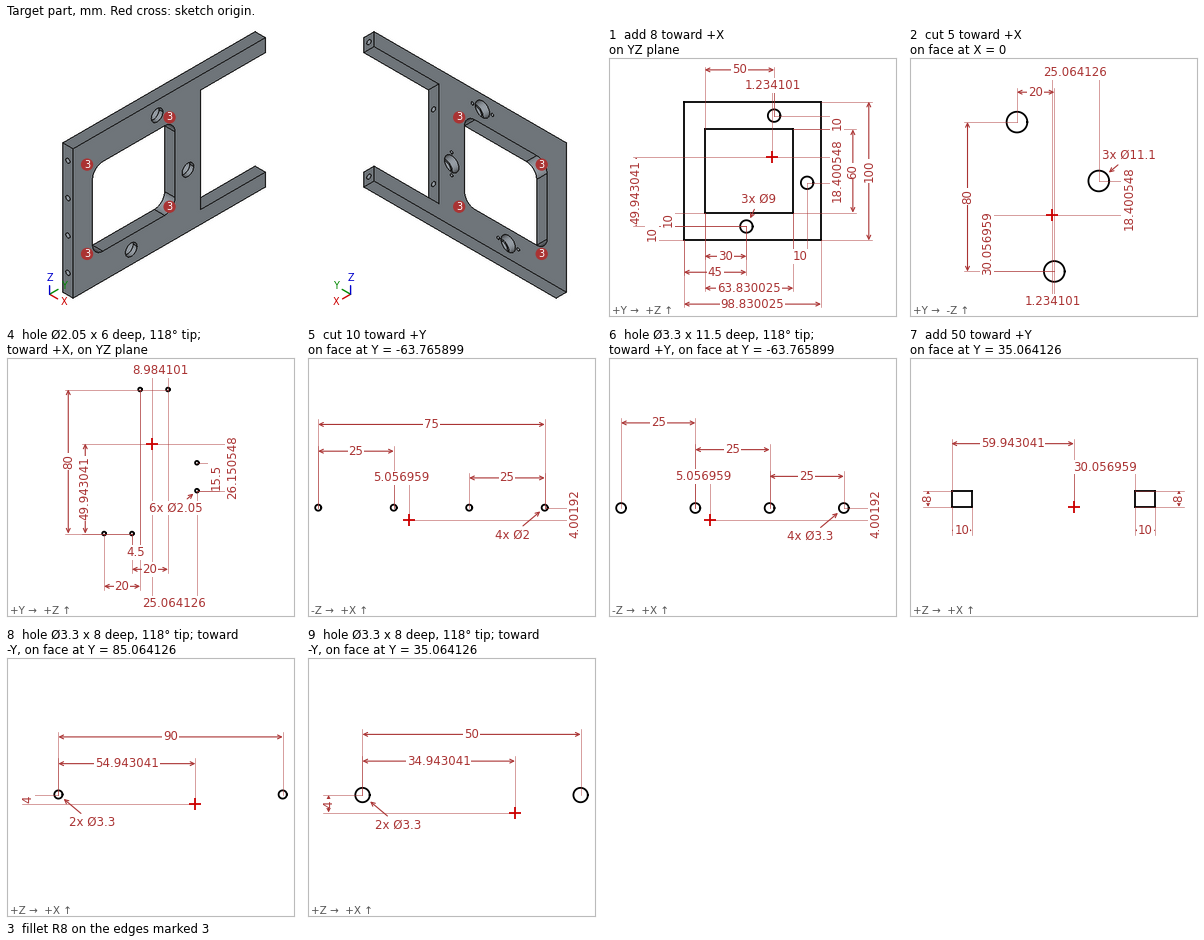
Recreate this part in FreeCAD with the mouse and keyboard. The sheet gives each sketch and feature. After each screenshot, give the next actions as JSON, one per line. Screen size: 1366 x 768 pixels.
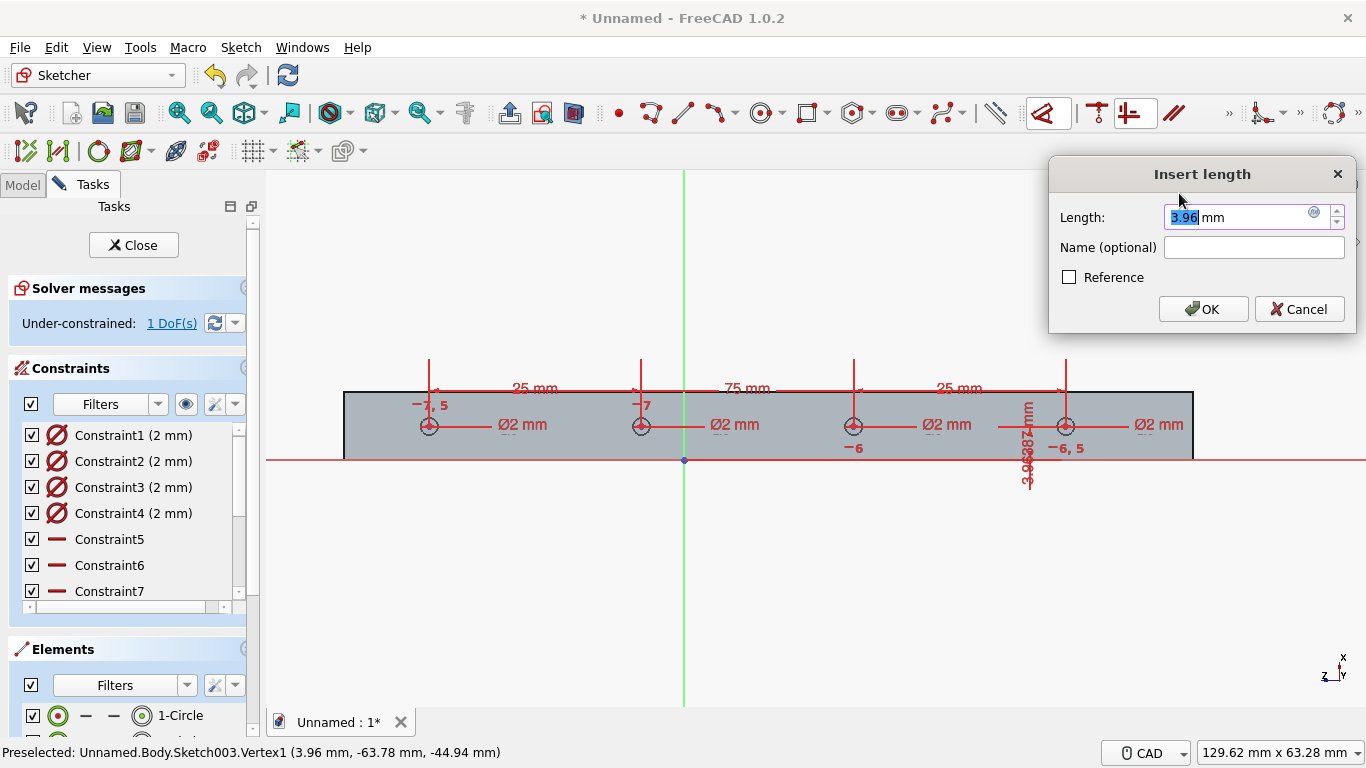
{"action": "type", "text": "4.00192"}
{"action": "key", "text": "Return"}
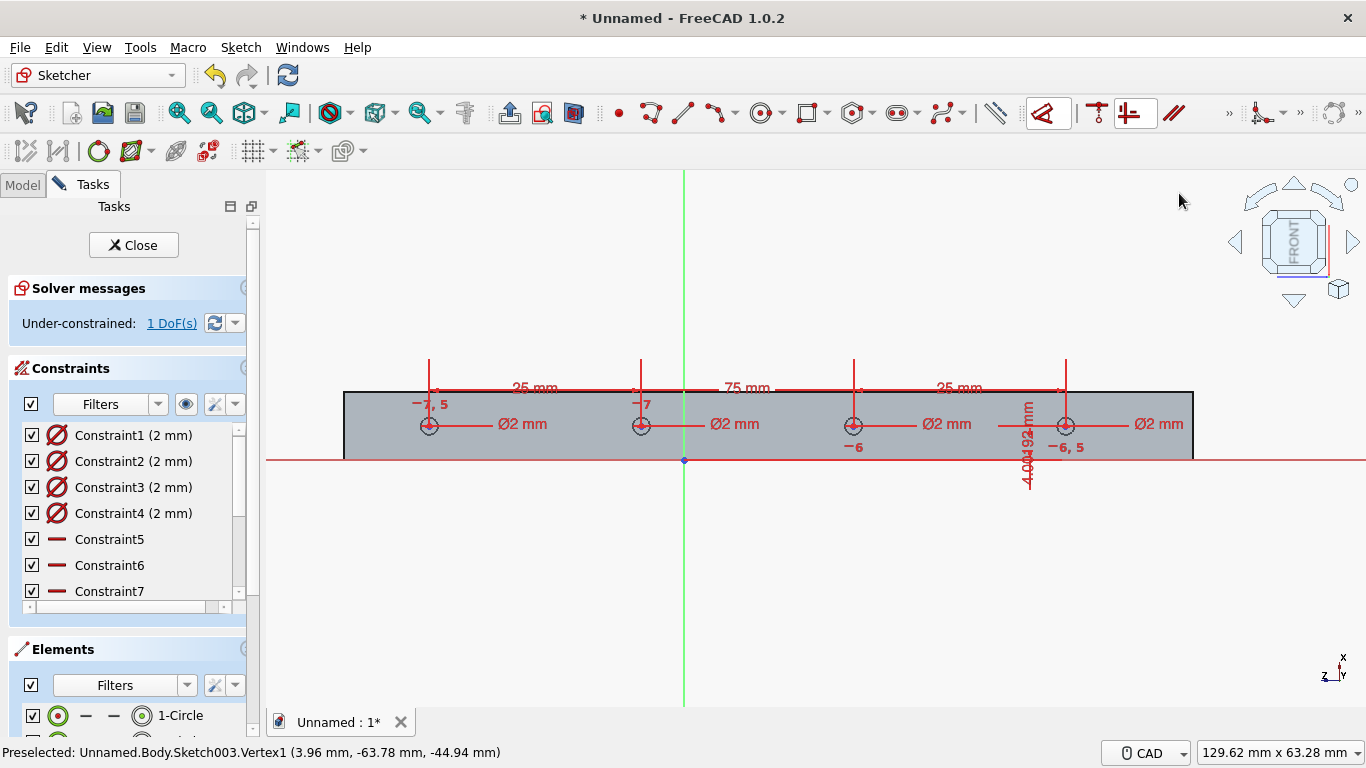
{"action": "left_click", "coordinate": [641, 426]}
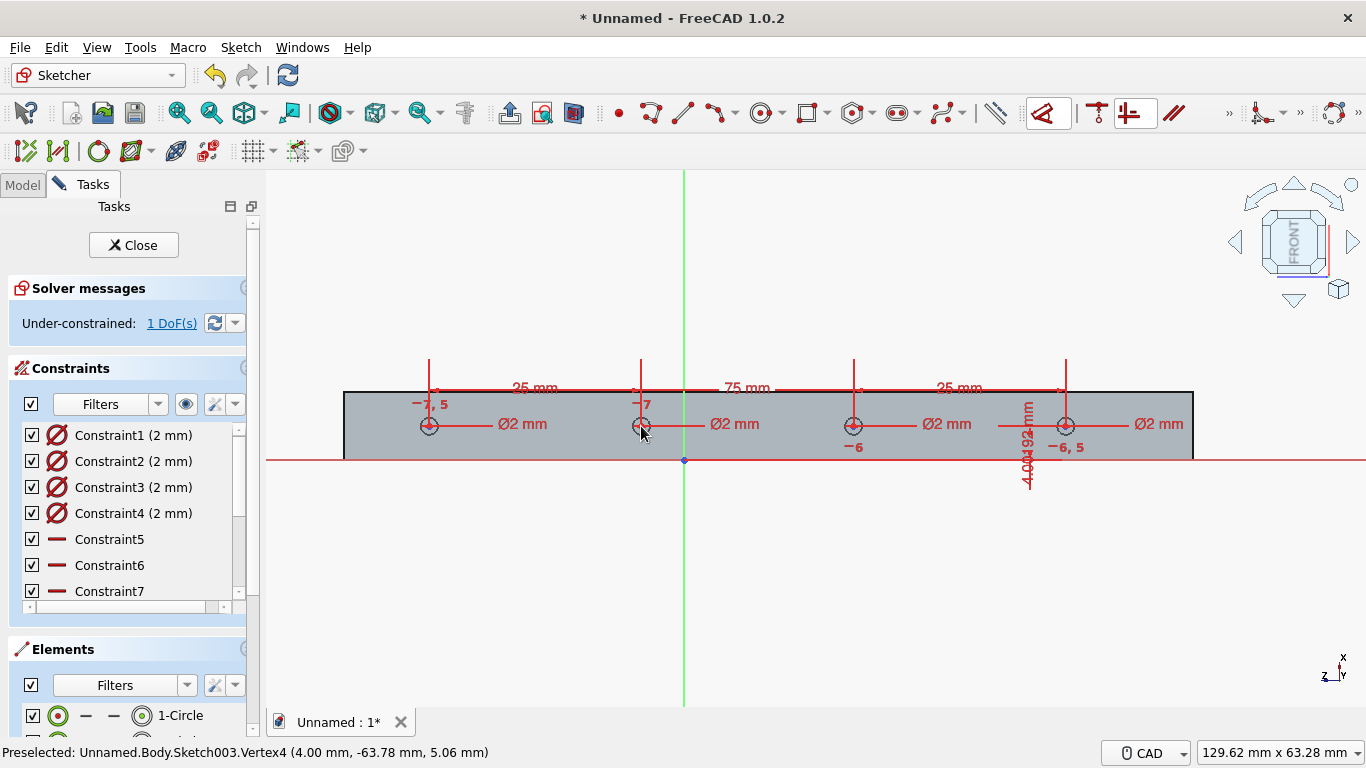
{"action": "key", "text": "l"}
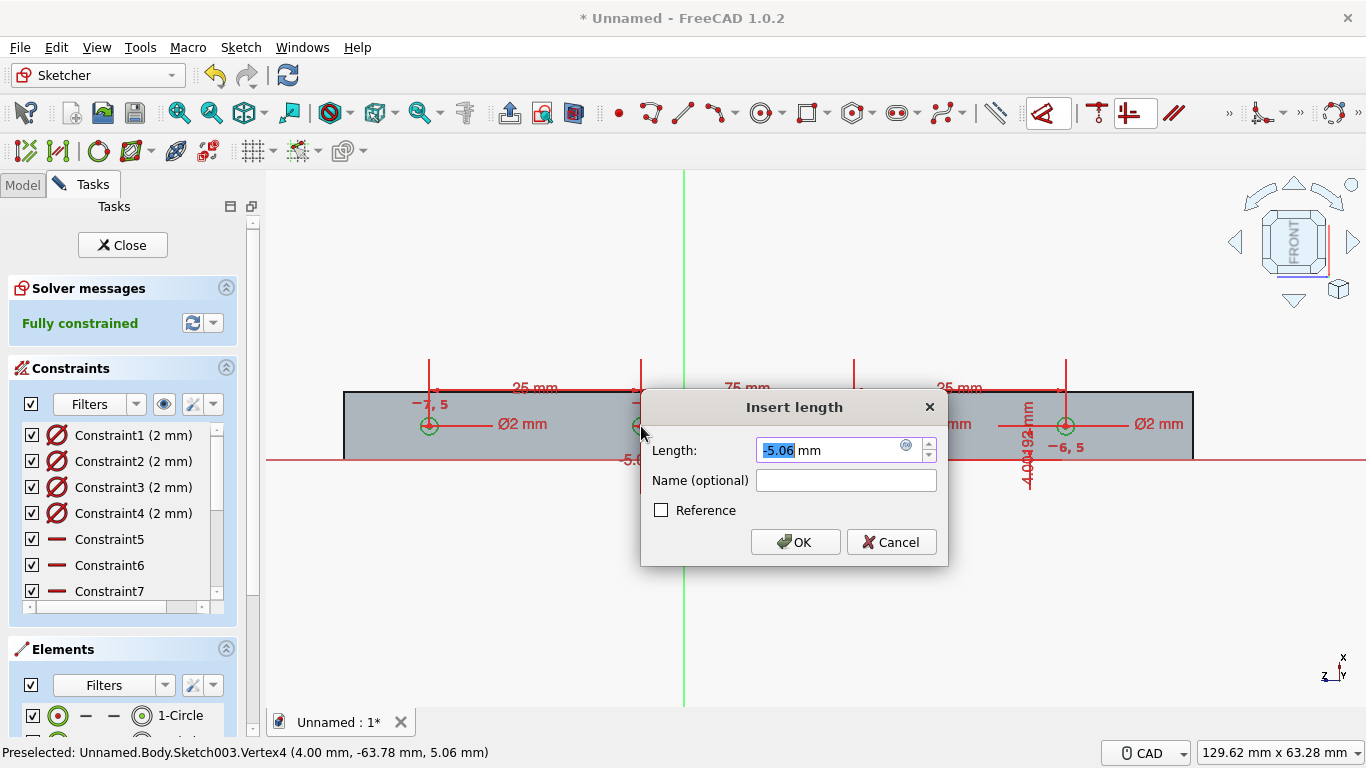
{"action": "type", "text": "-5.056959"}
{"action": "key", "text": "Return"}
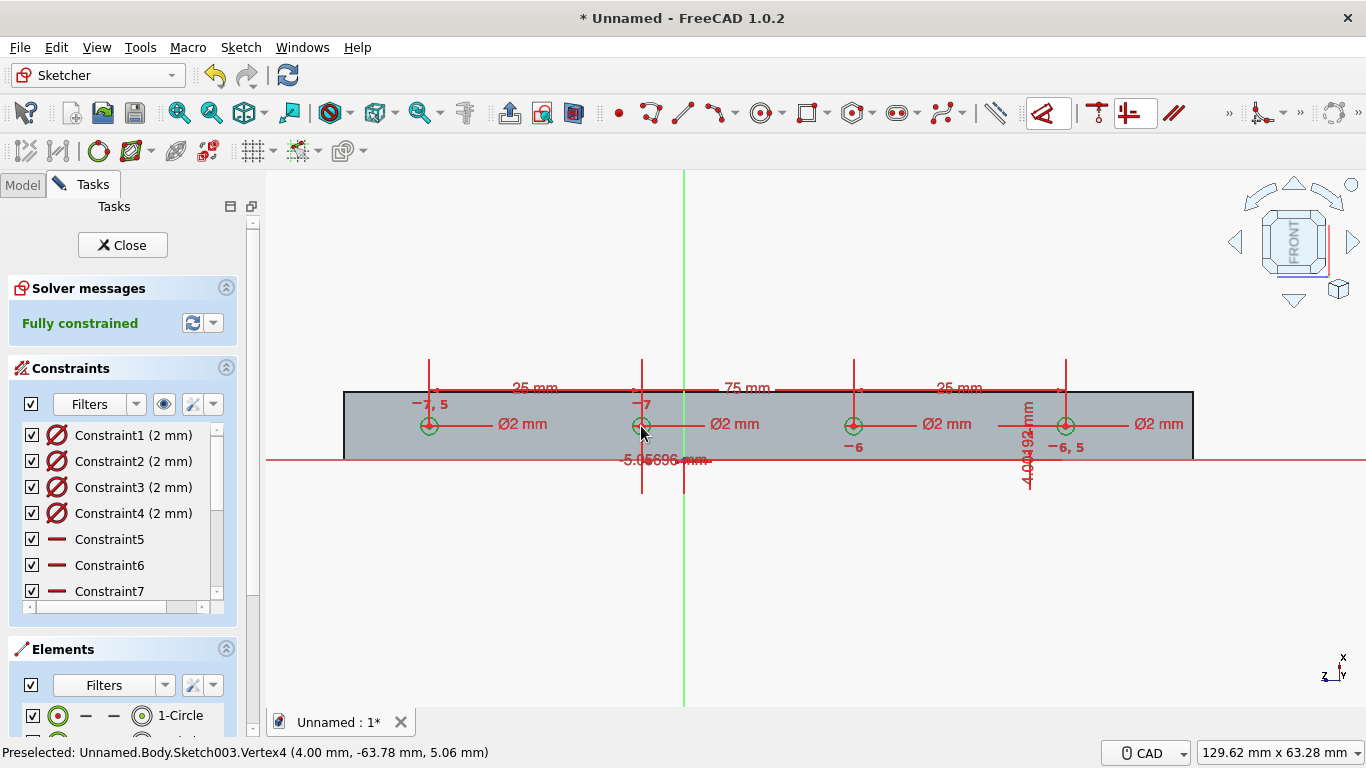
{"action": "left_click", "coordinate": [123, 245]}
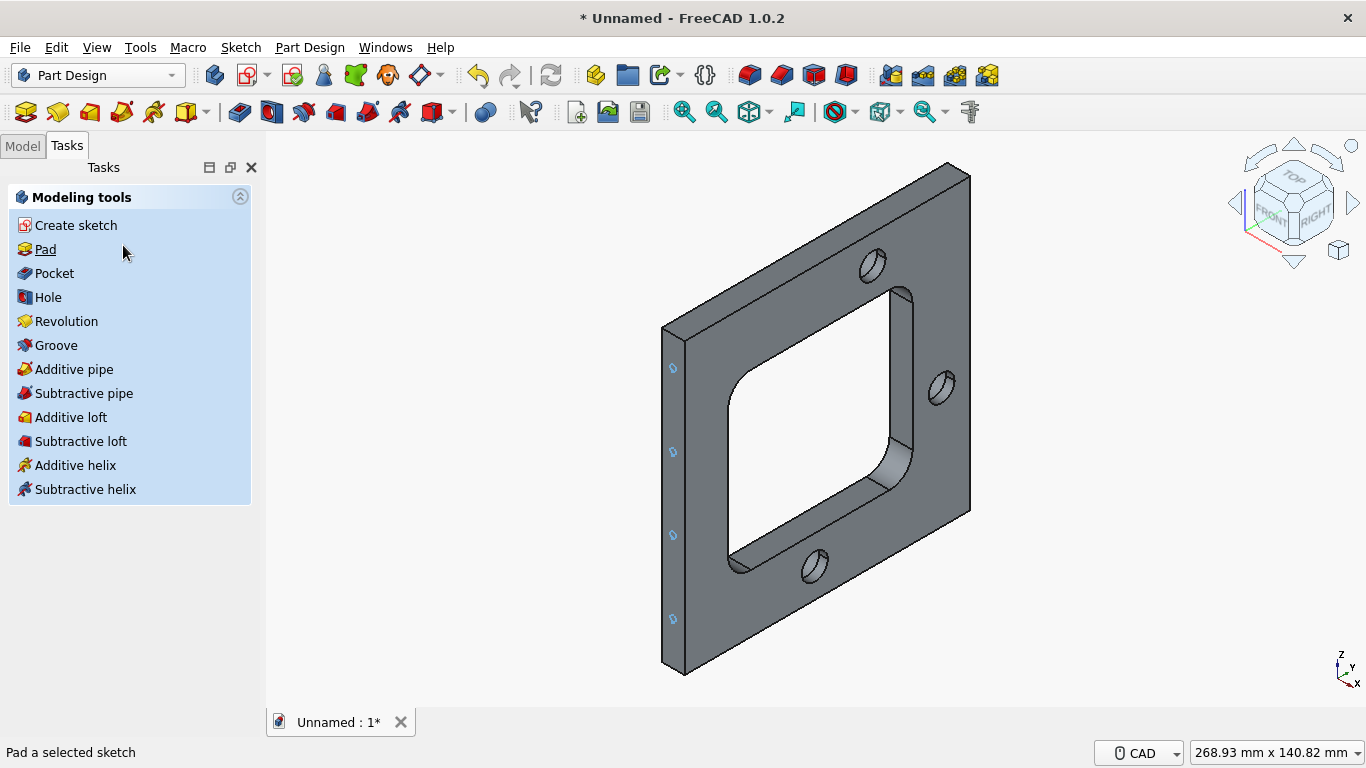
{"action": "left_click", "coordinate": [240, 112]}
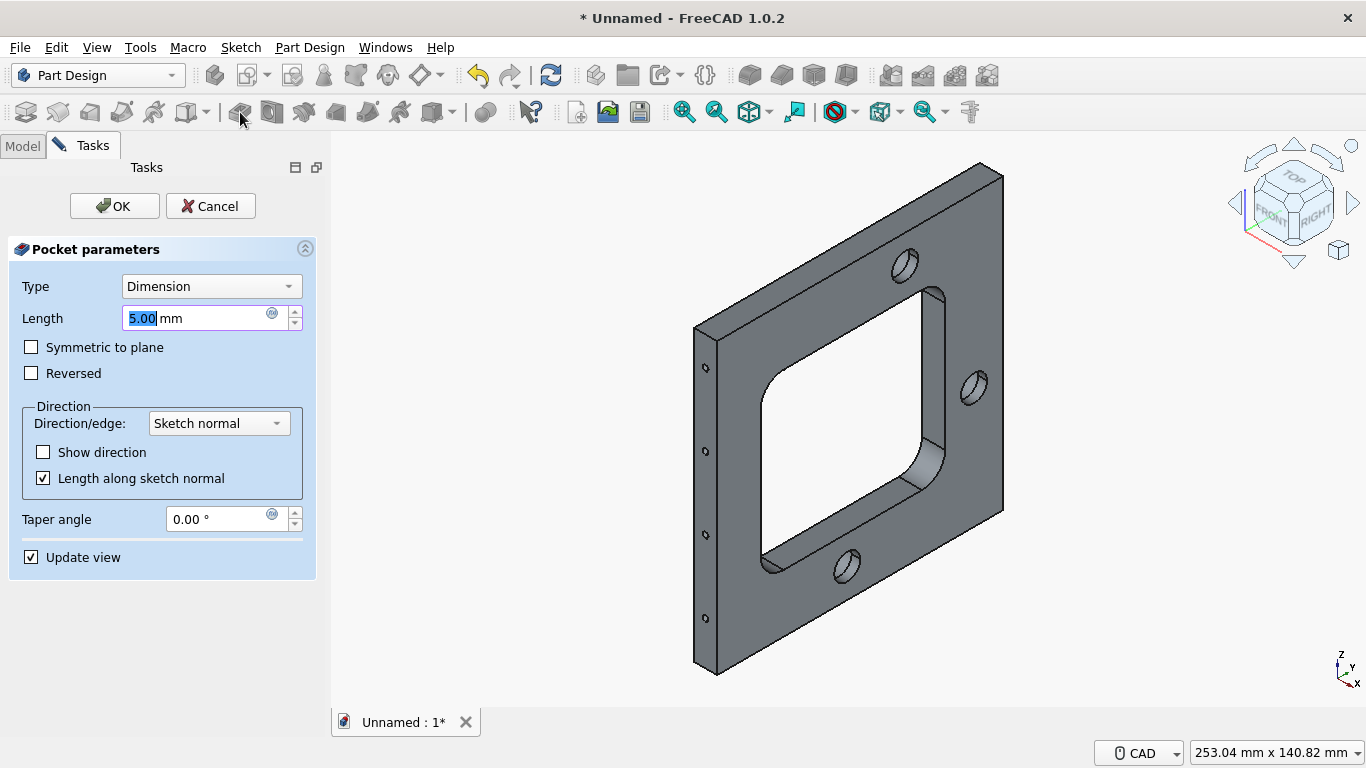
{"action": "type", "text": "10"}
{"action": "key", "text": "Tab"}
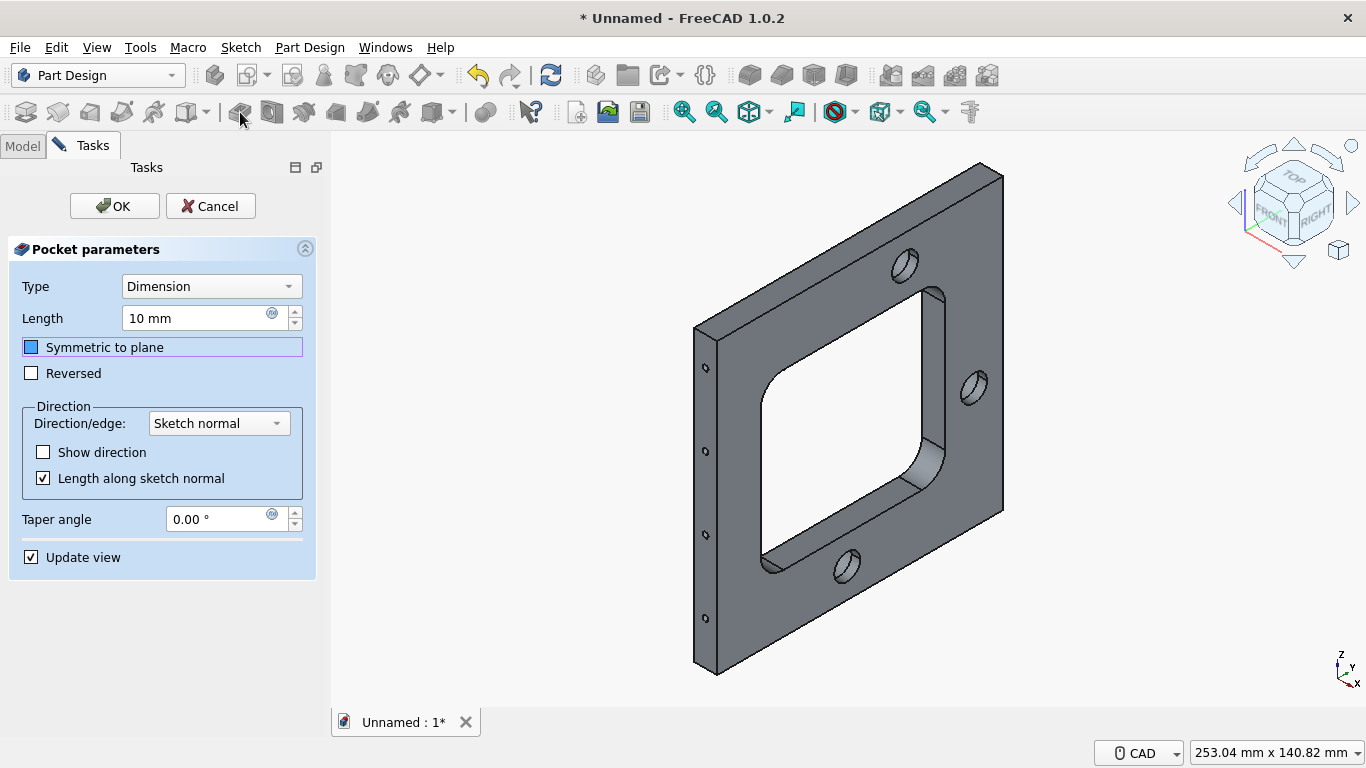
{"action": "left_click", "coordinate": [115, 206]}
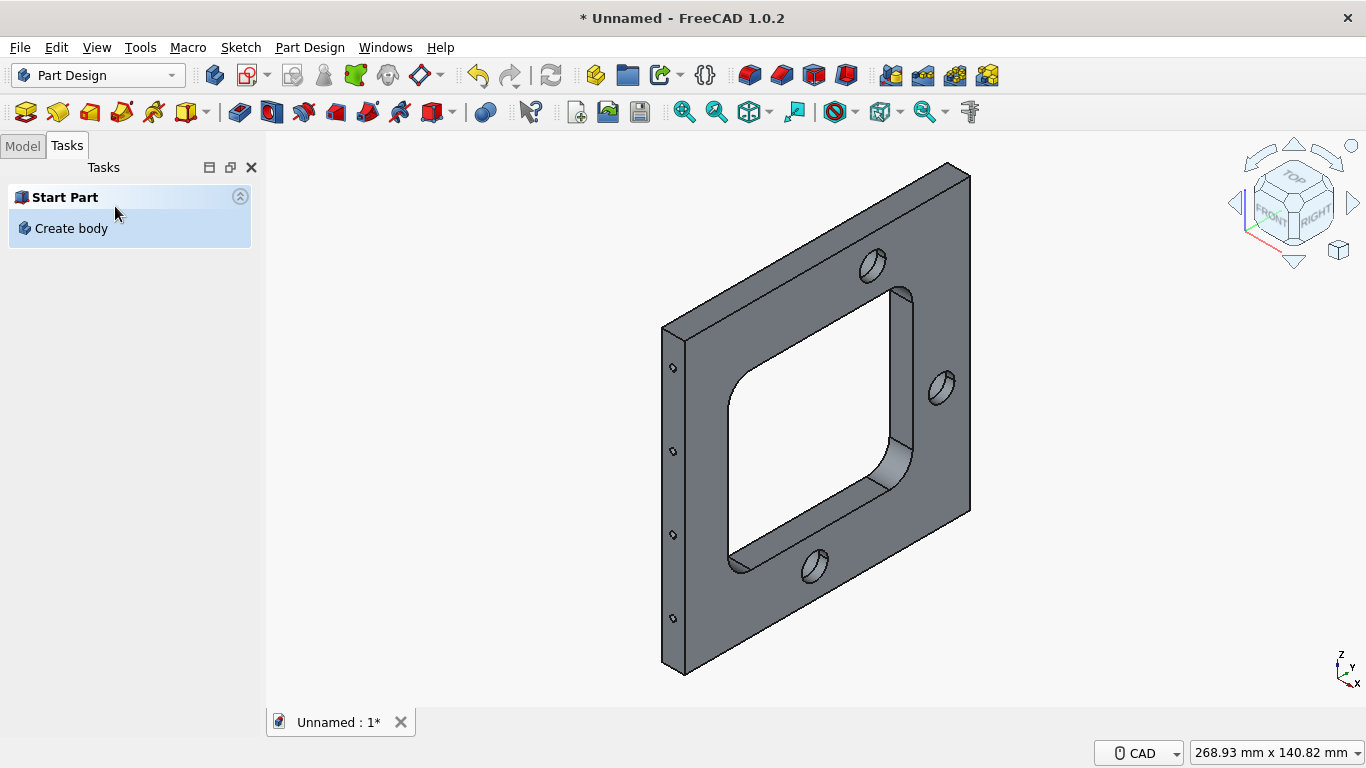
{"action": "left_click", "coordinate": [673, 644]}